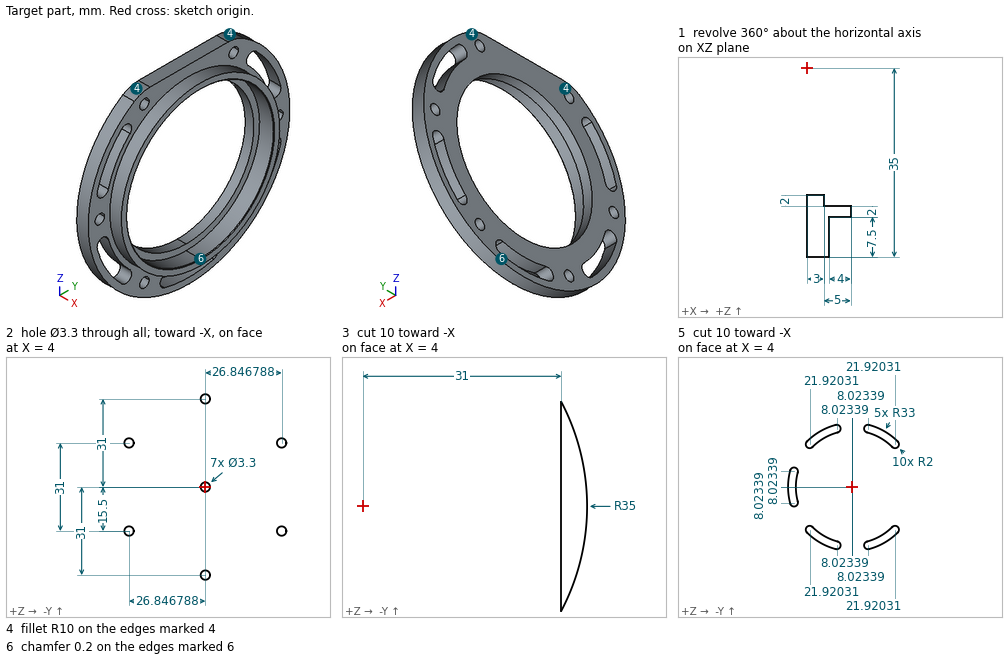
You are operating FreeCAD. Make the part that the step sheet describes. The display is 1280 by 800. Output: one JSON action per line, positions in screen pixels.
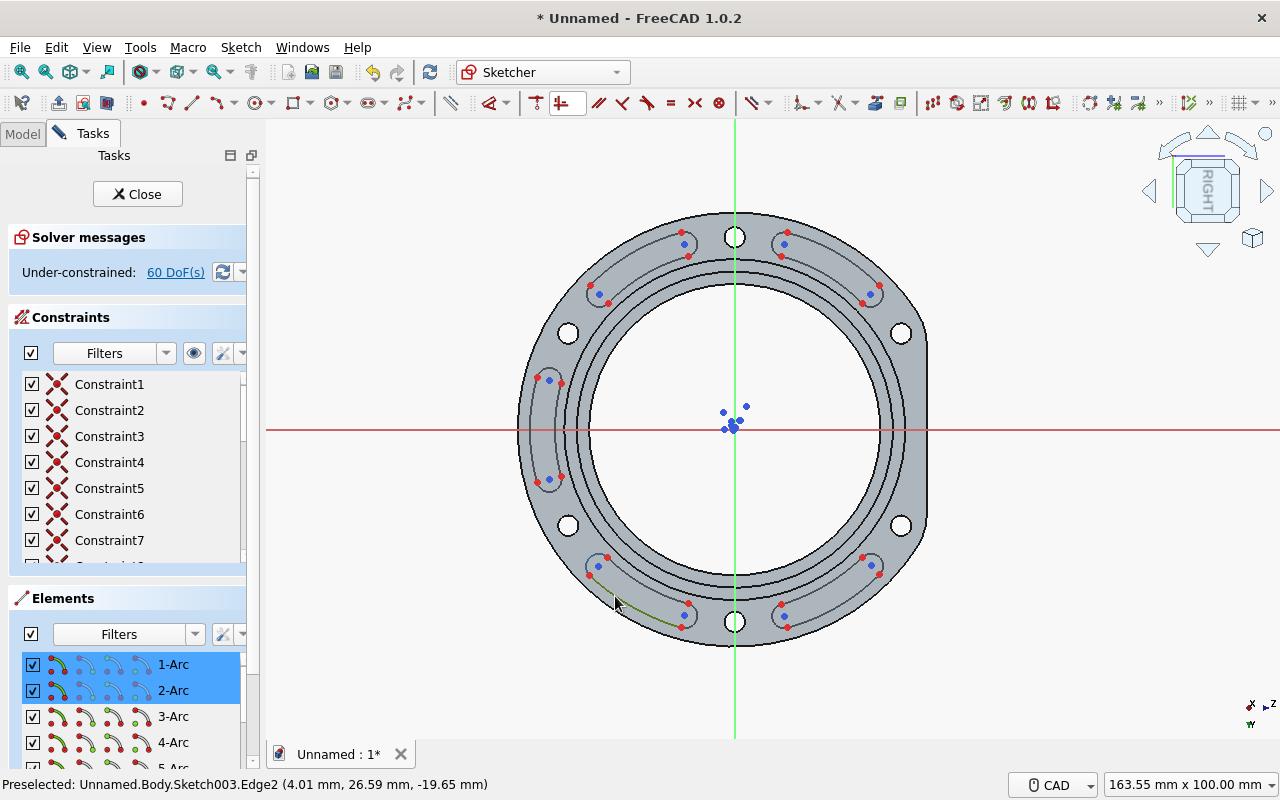
{"action": "left_click", "coordinate": [648, 104]}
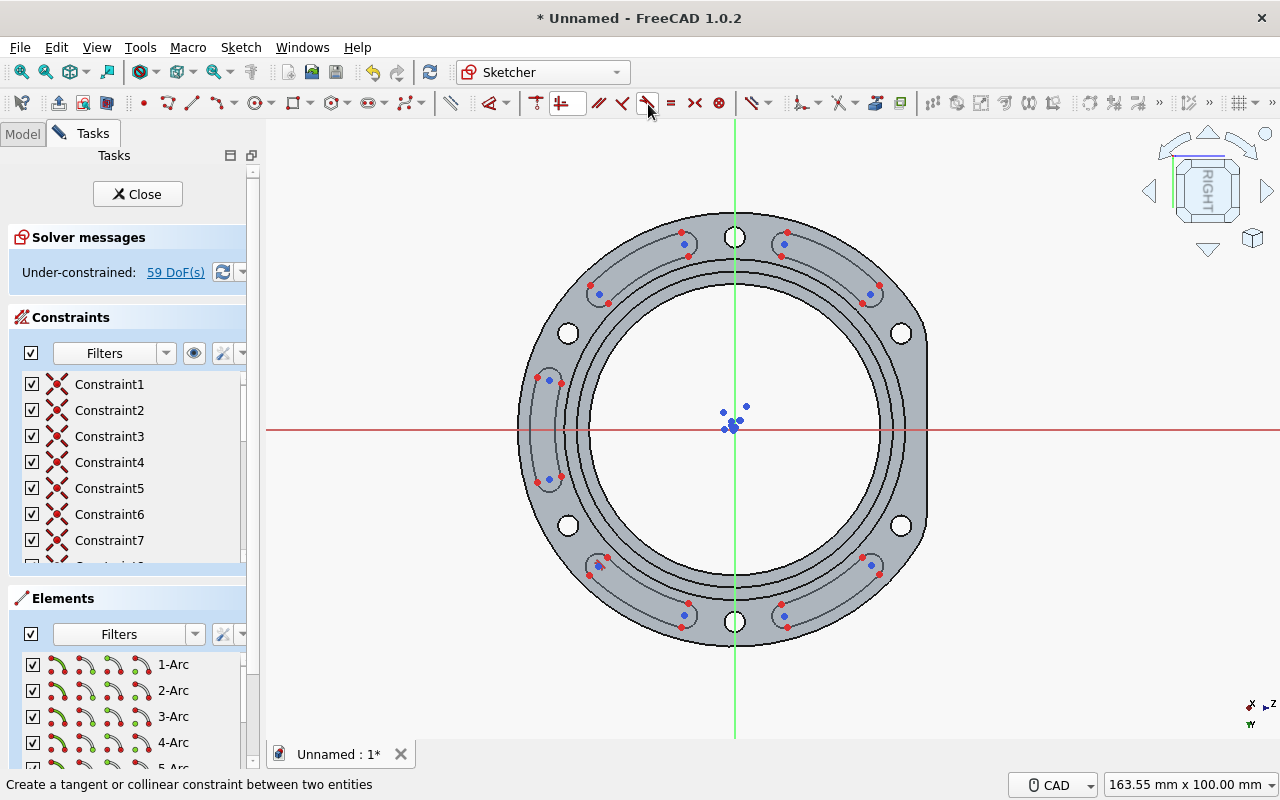
{"action": "left_click", "coordinate": [597, 554]}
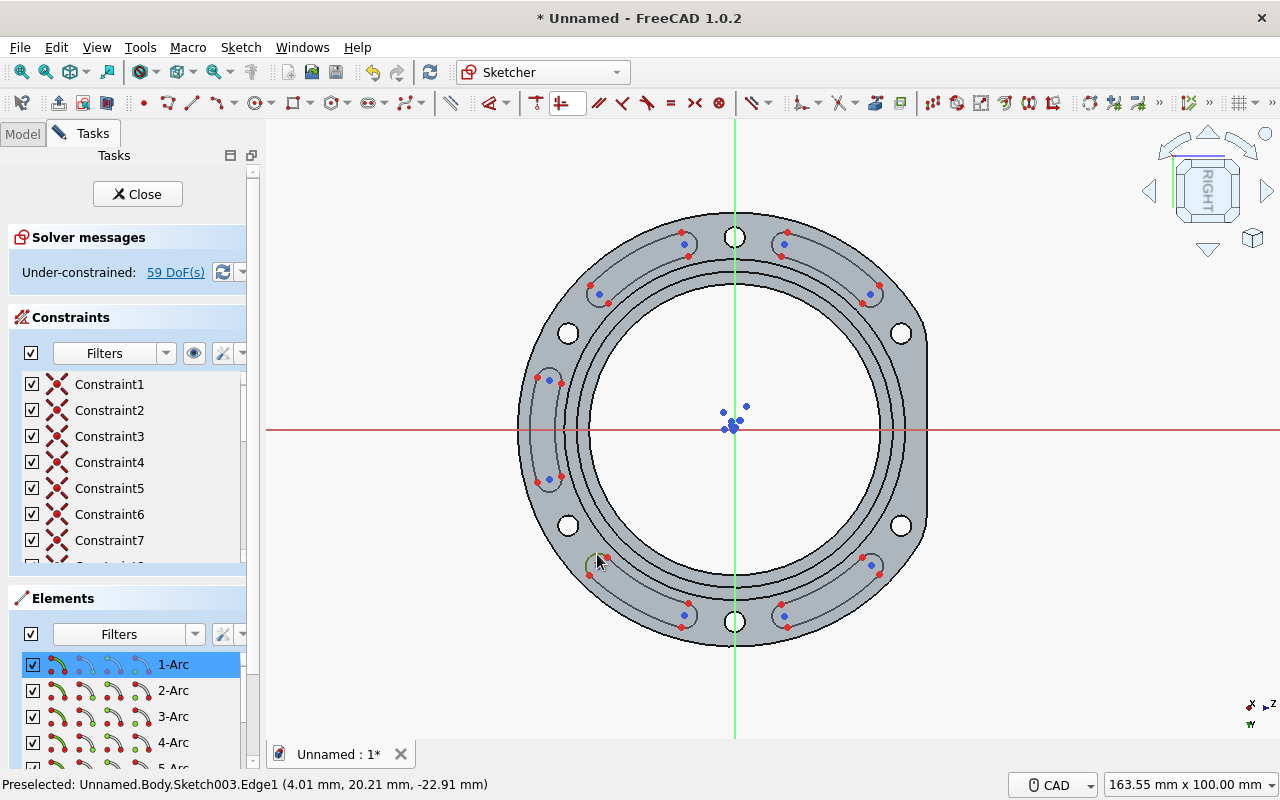
{"action": "left_click", "coordinate": [629, 576]}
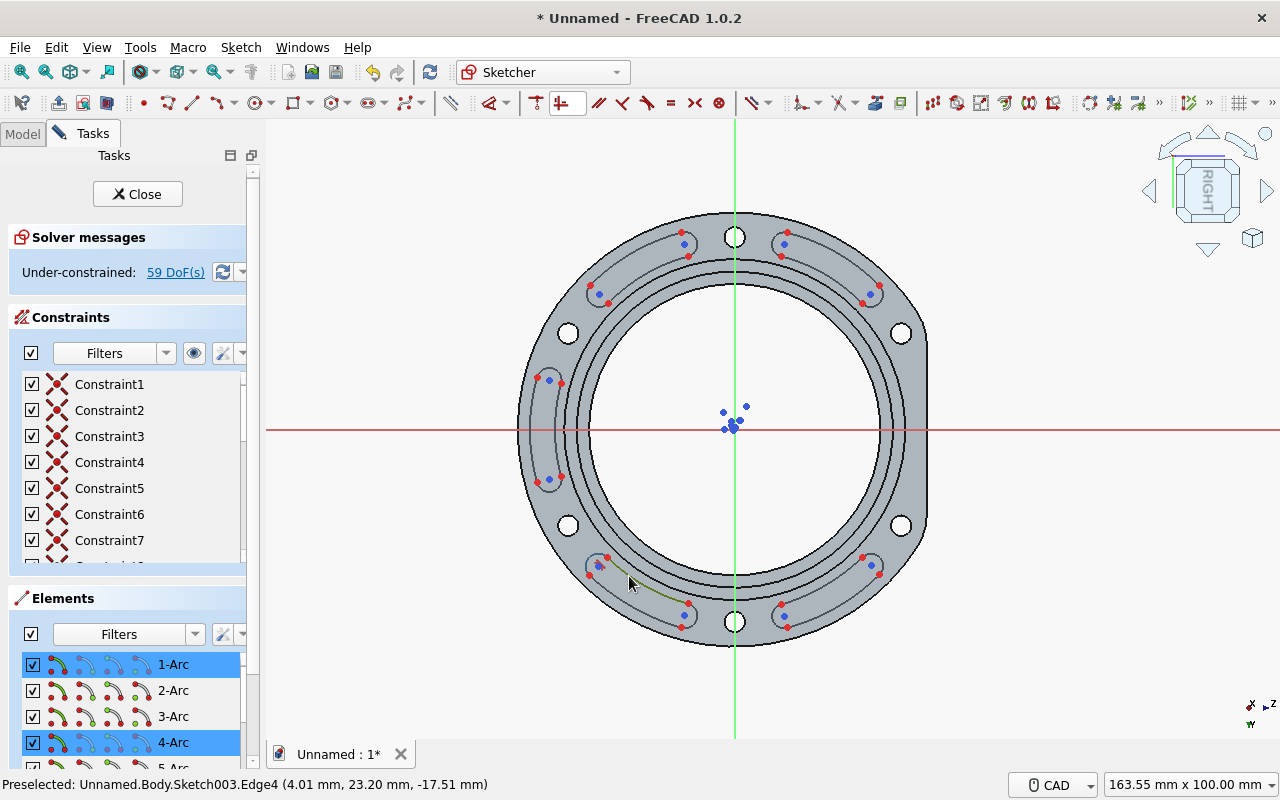
{"action": "left_click", "coordinate": [648, 104]}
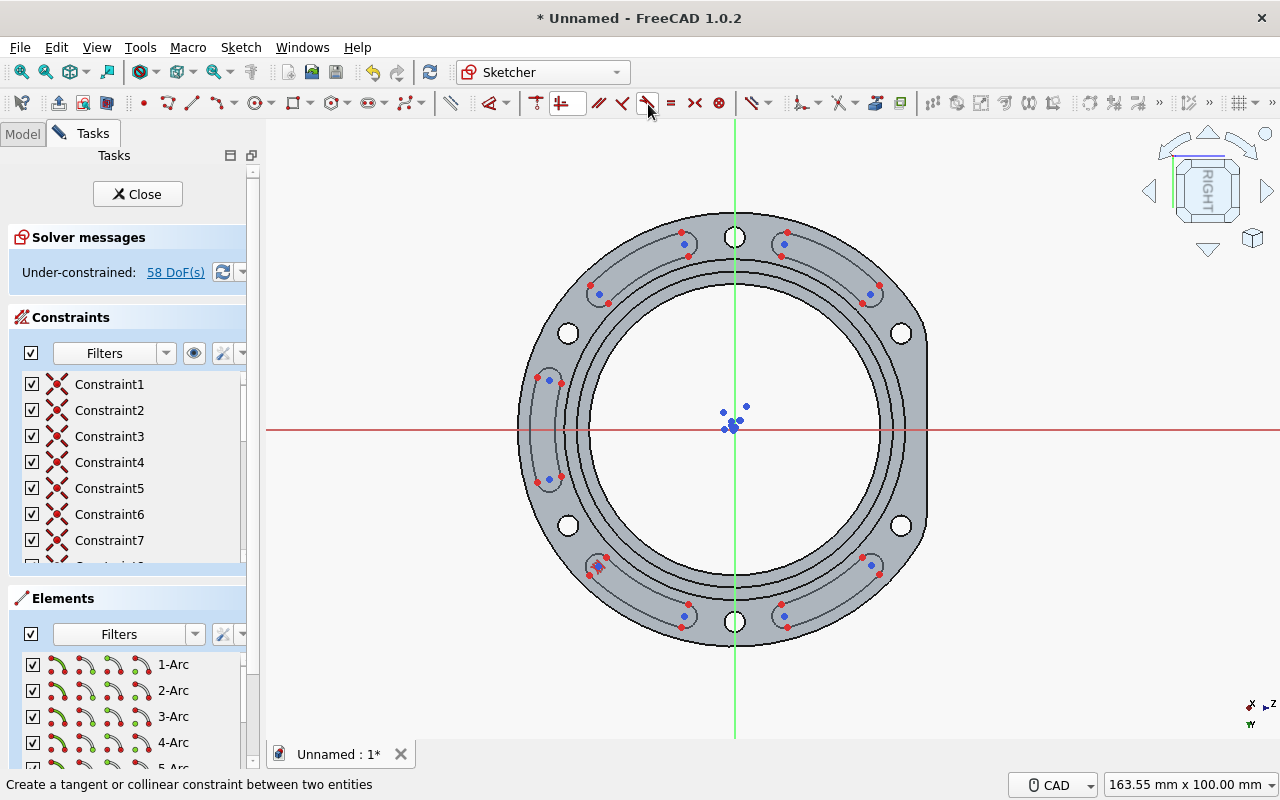
{"action": "left_click", "coordinate": [615, 596]}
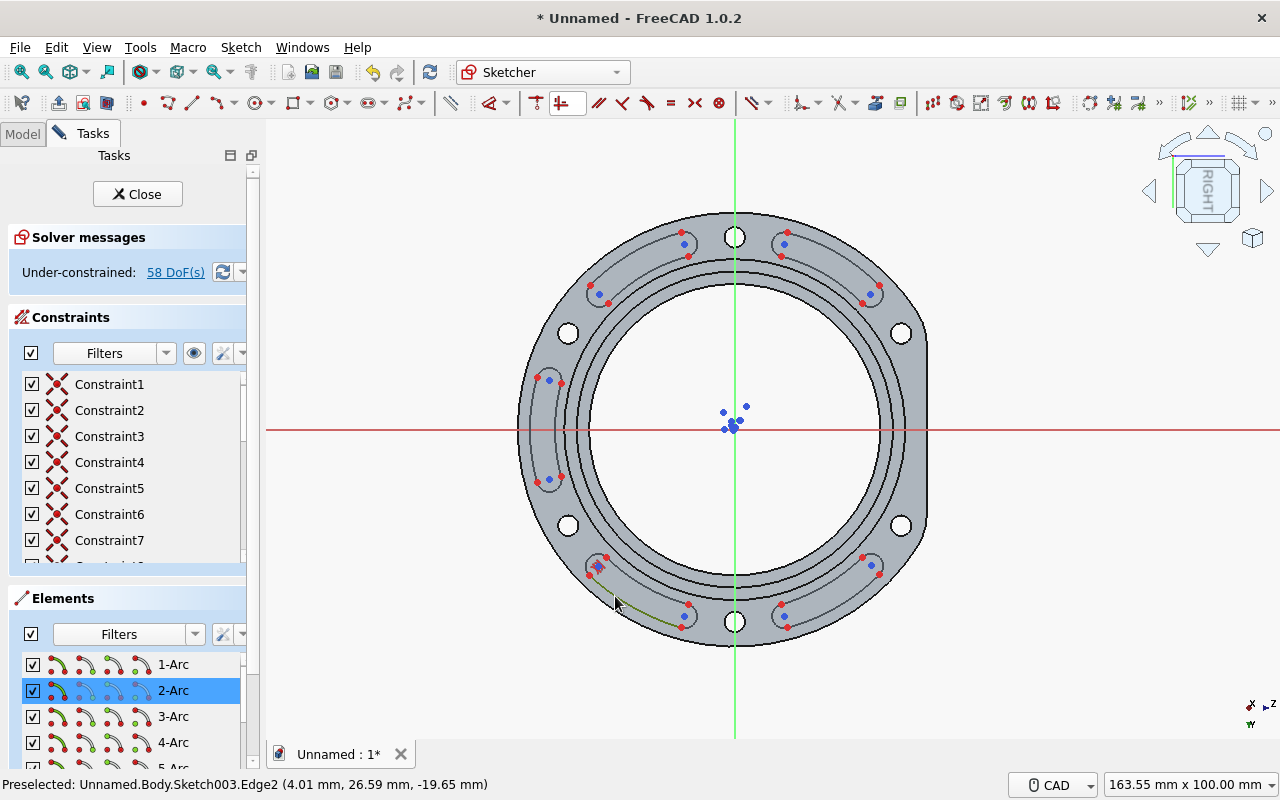
{"action": "scroll", "coordinate": [692, 626], "scroll_direction": "up", "scroll_amount": 2}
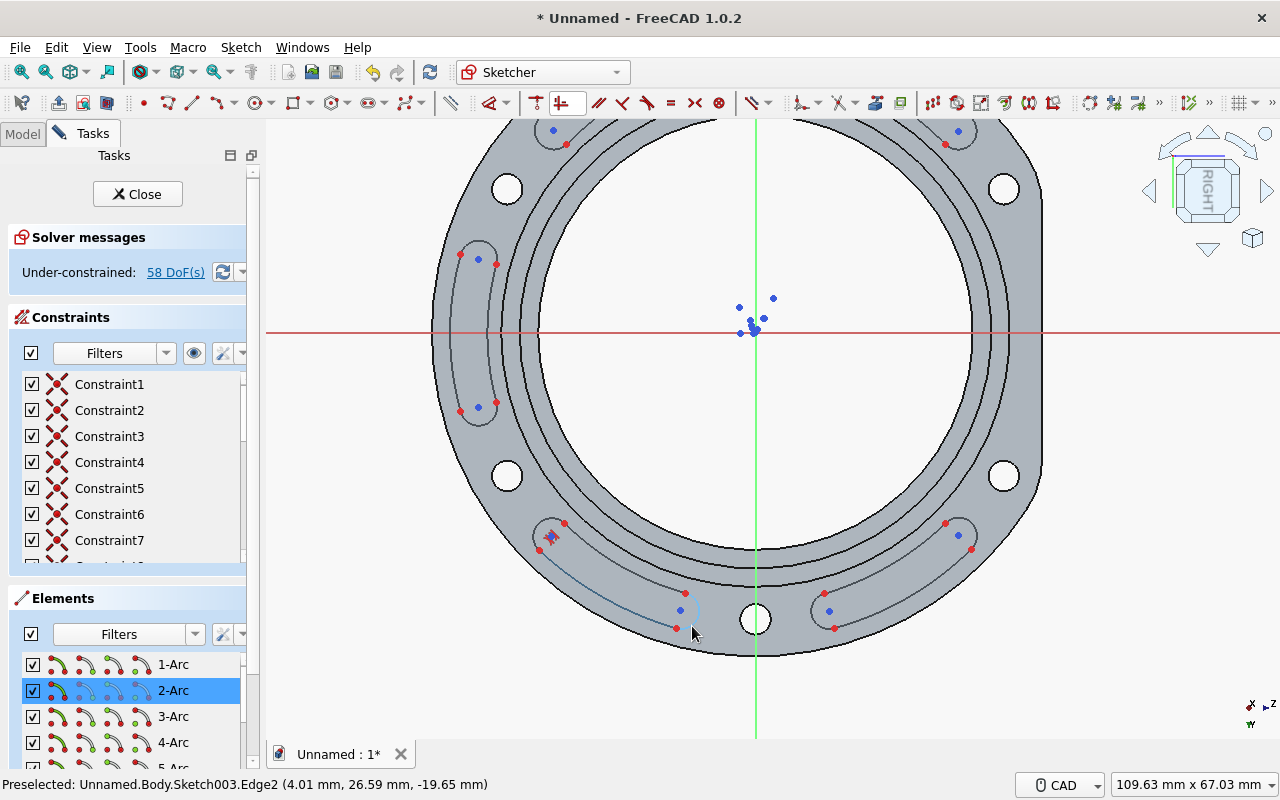
{"action": "left_click", "coordinate": [693, 625]}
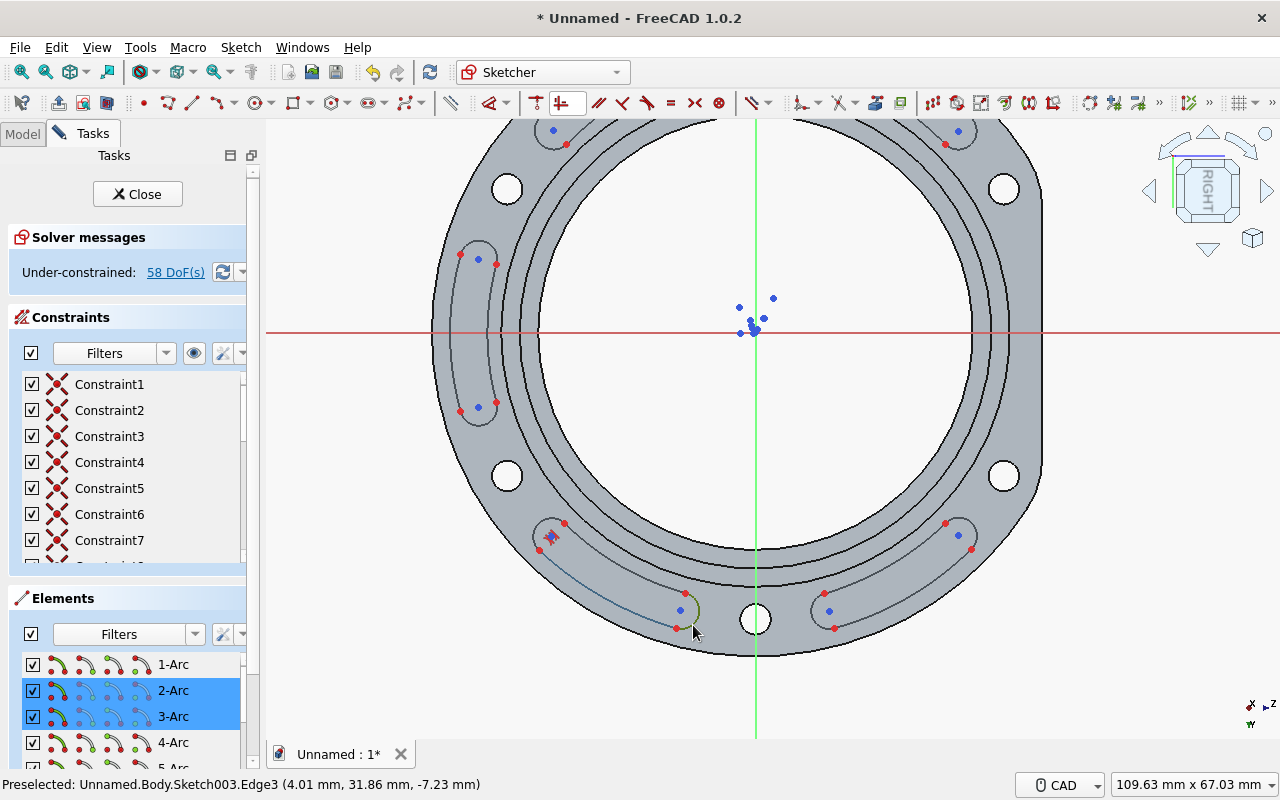
{"action": "left_click", "coordinate": [648, 104]}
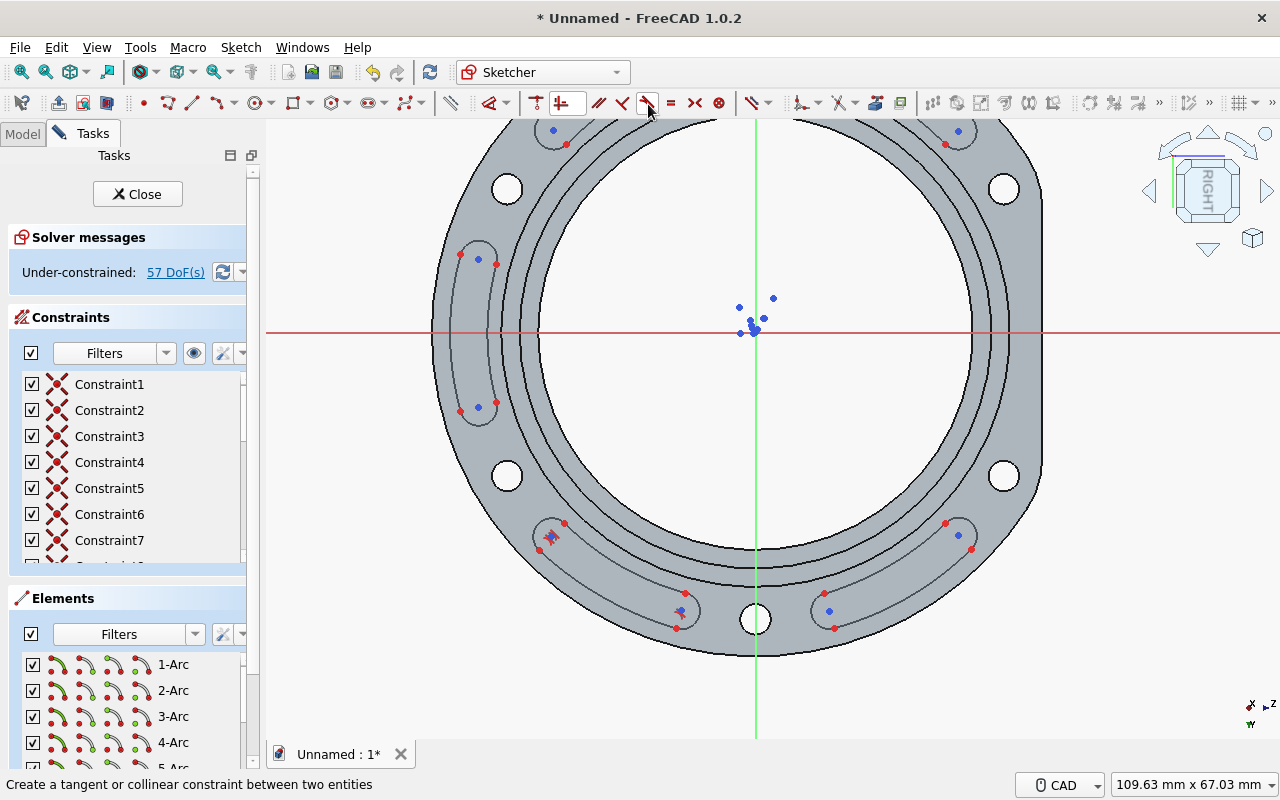
{"action": "left_click", "coordinate": [693, 625]}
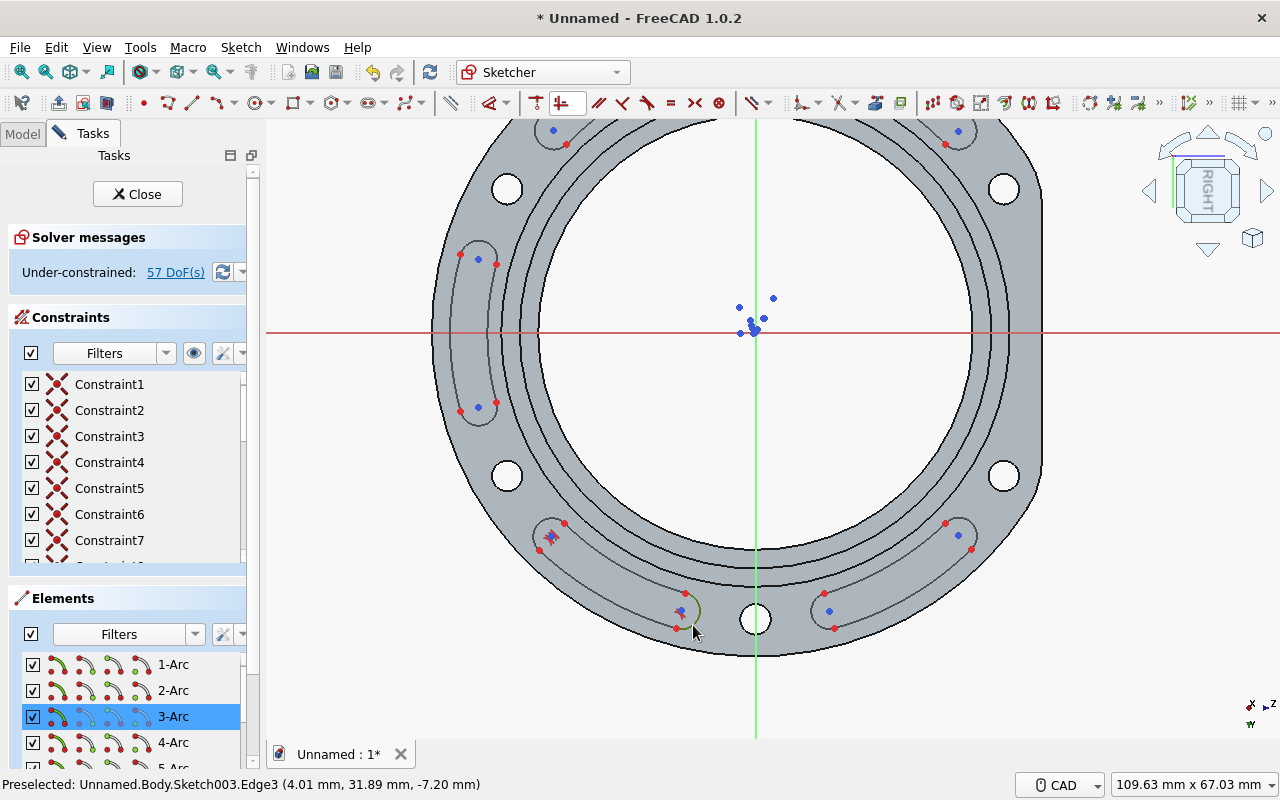
{"action": "left_click", "coordinate": [597, 551]}